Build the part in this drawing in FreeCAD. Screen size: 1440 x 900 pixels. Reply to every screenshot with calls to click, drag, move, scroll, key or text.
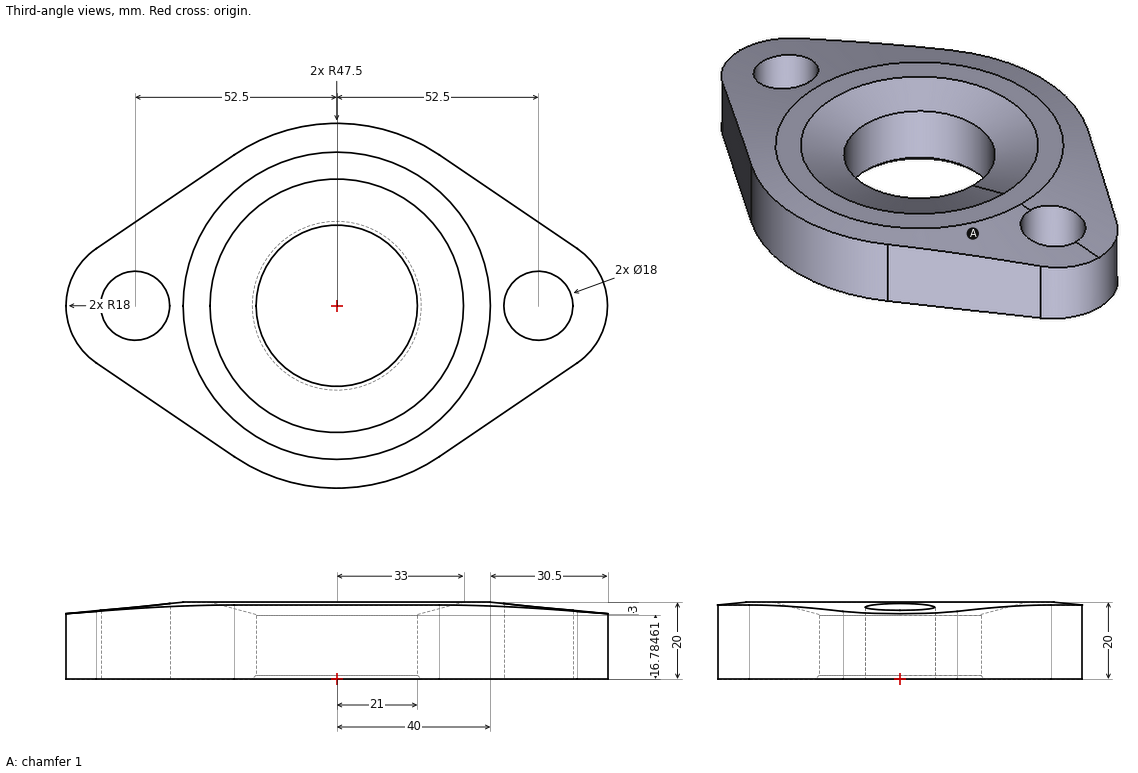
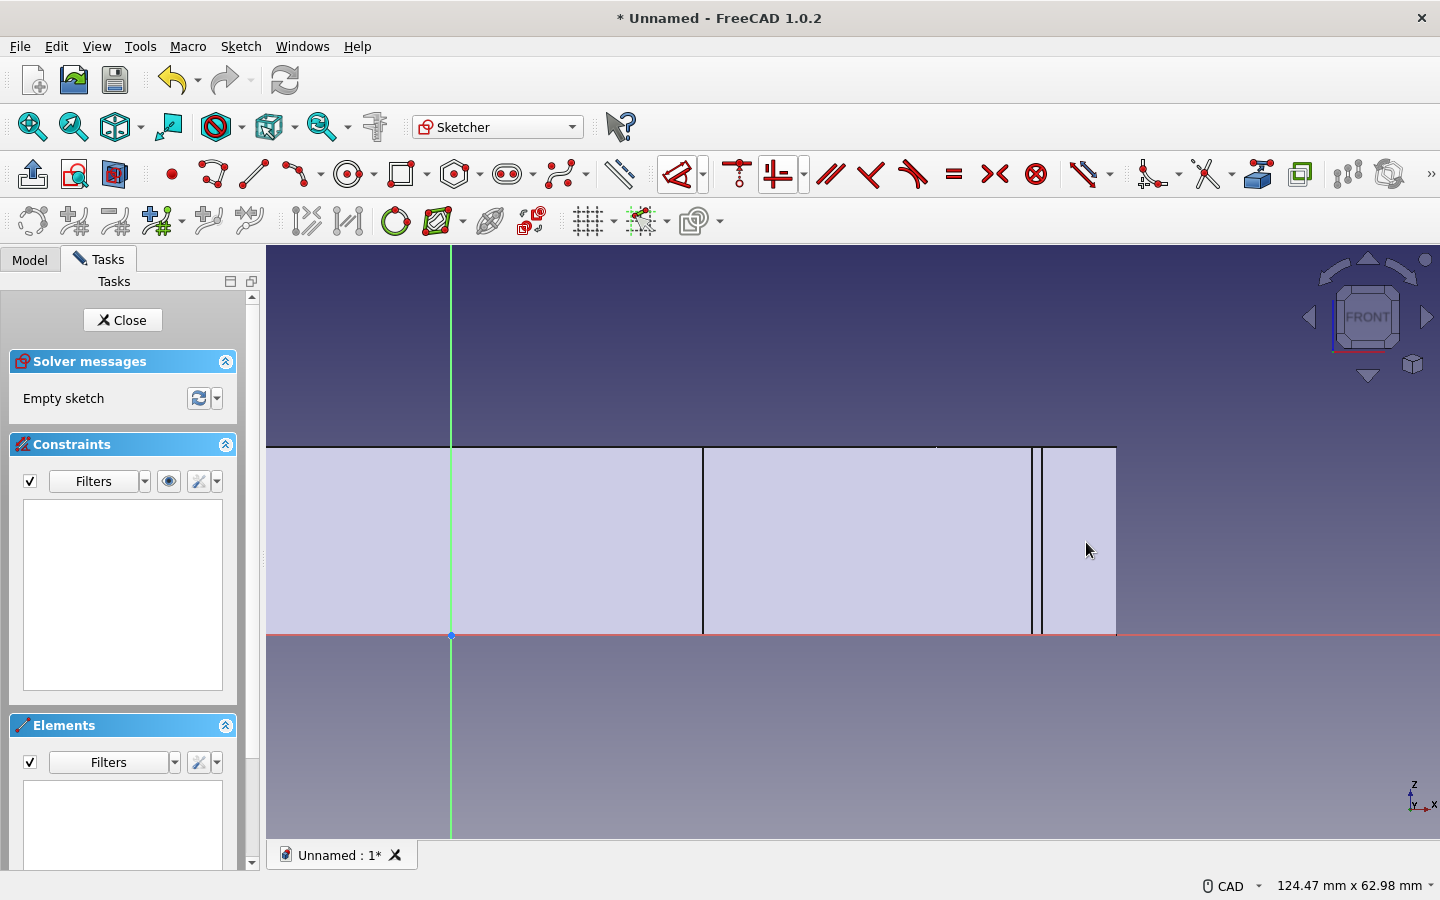
key(g)
key(m)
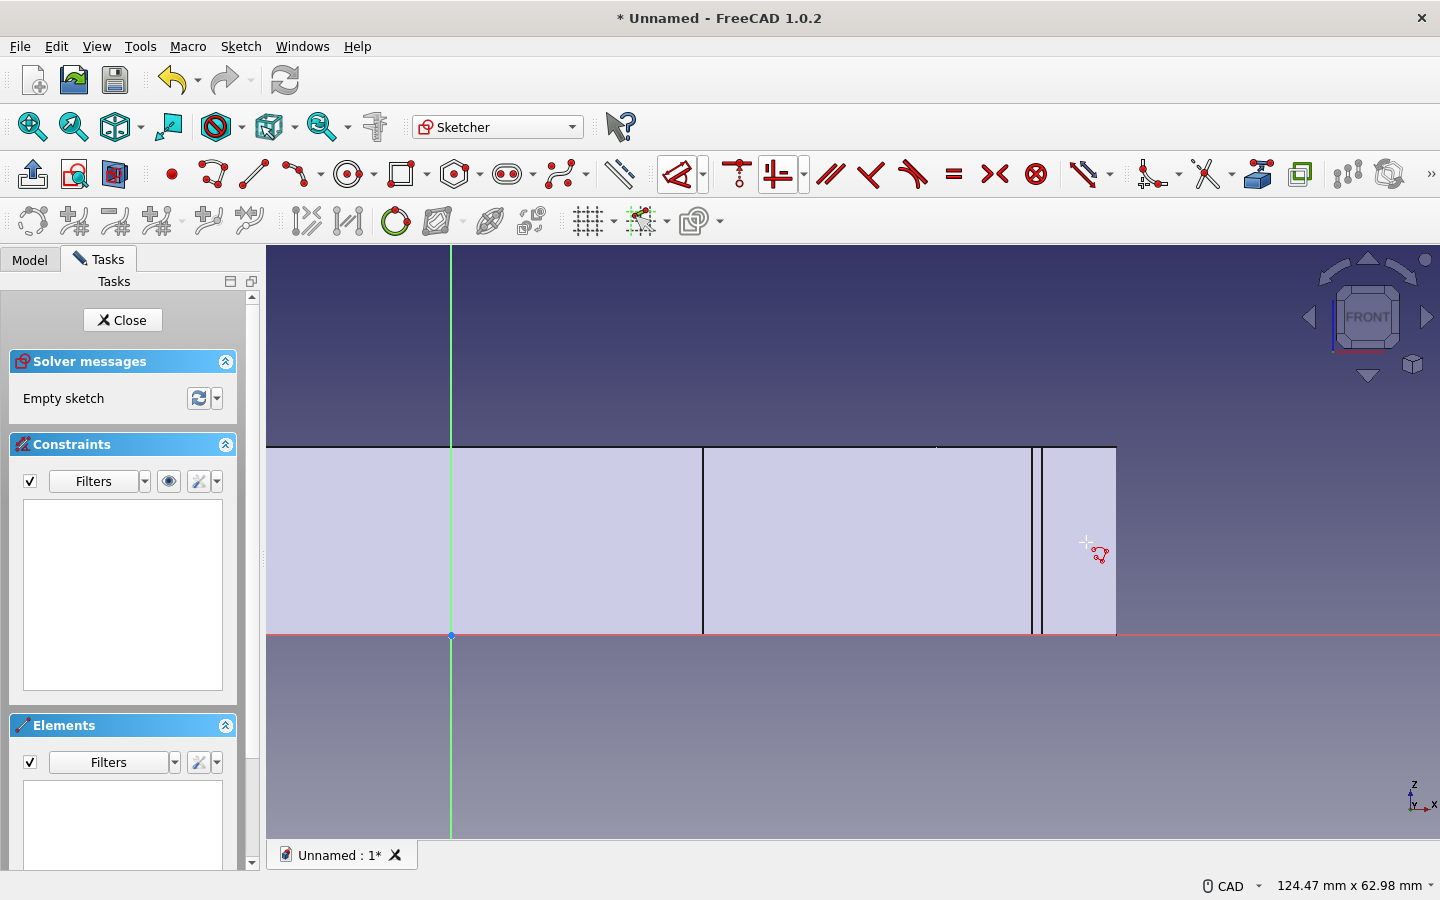
click(451, 635)
click(460, 447)
click(763, 447)
click(650, 477)
click(650, 626)
click(451, 635)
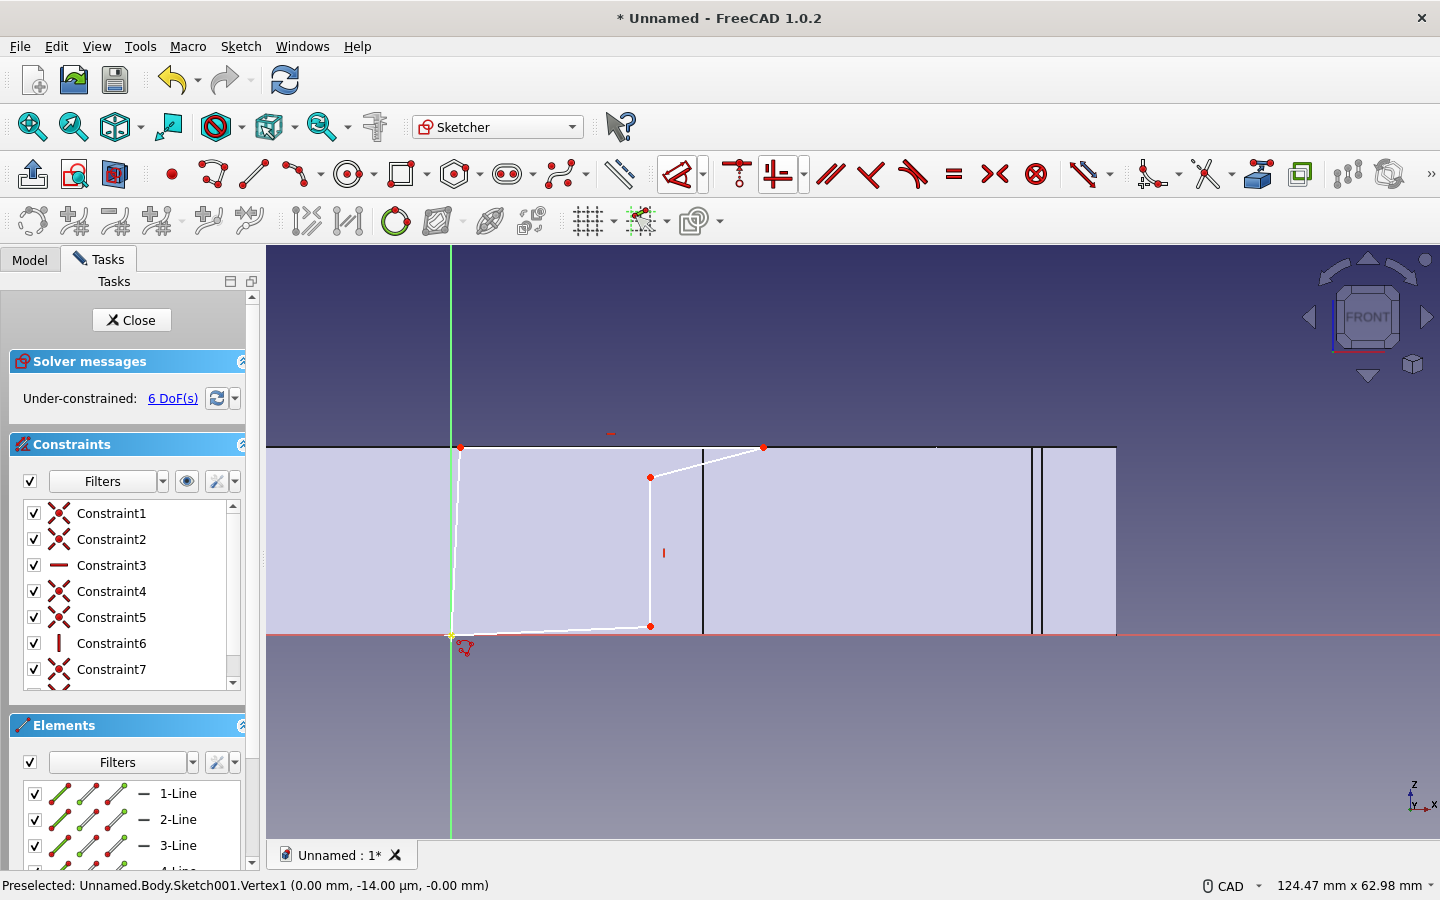
click(829, 447)
click(1116, 447)
click(1116, 475)
click(829, 448)
key(Escape)
key(Escape)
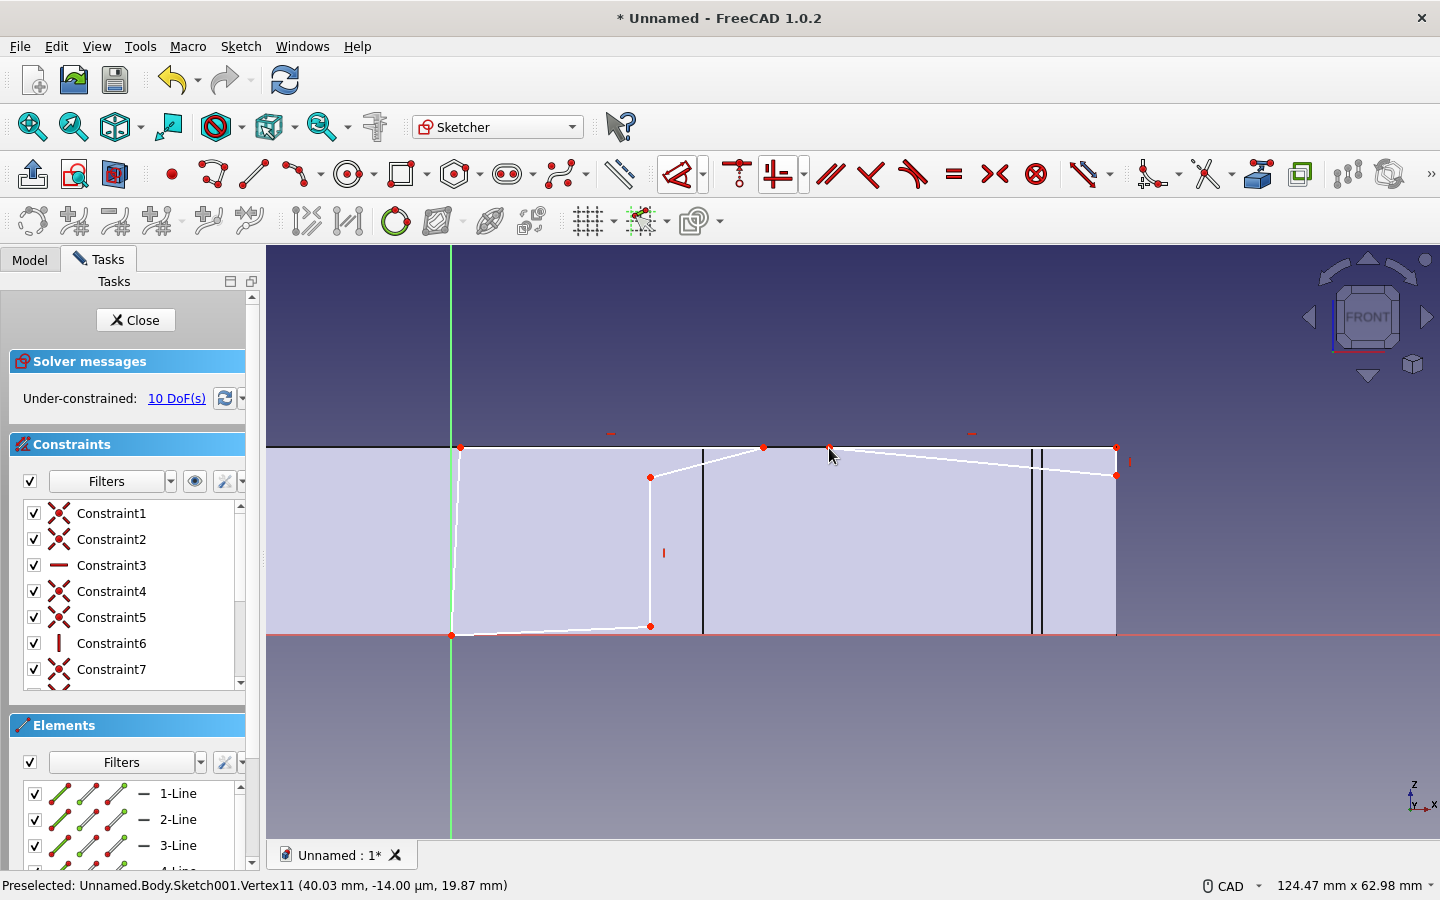
click(454, 579)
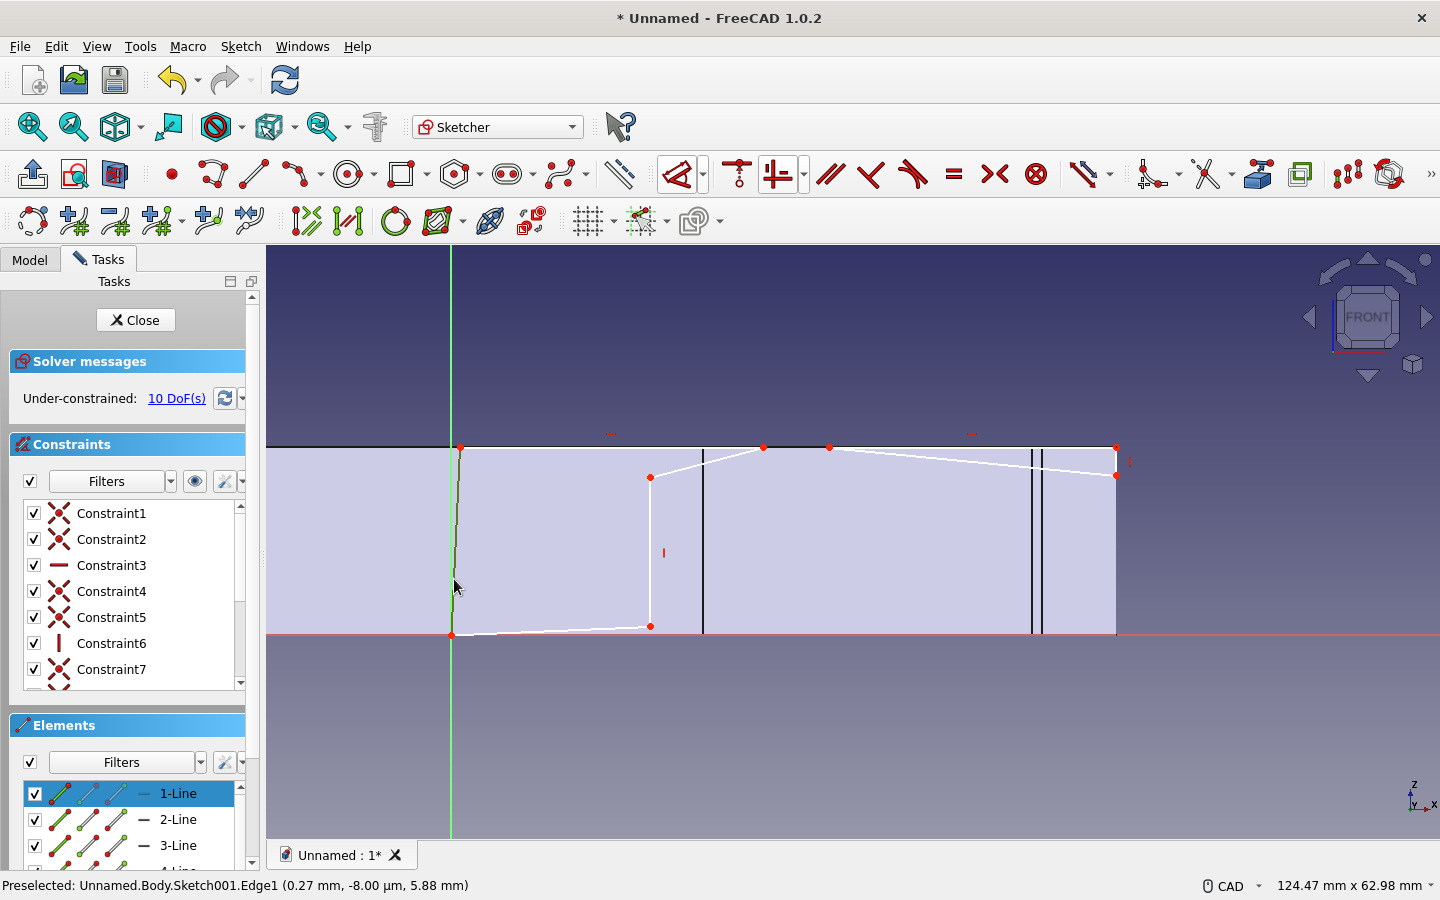
key(v)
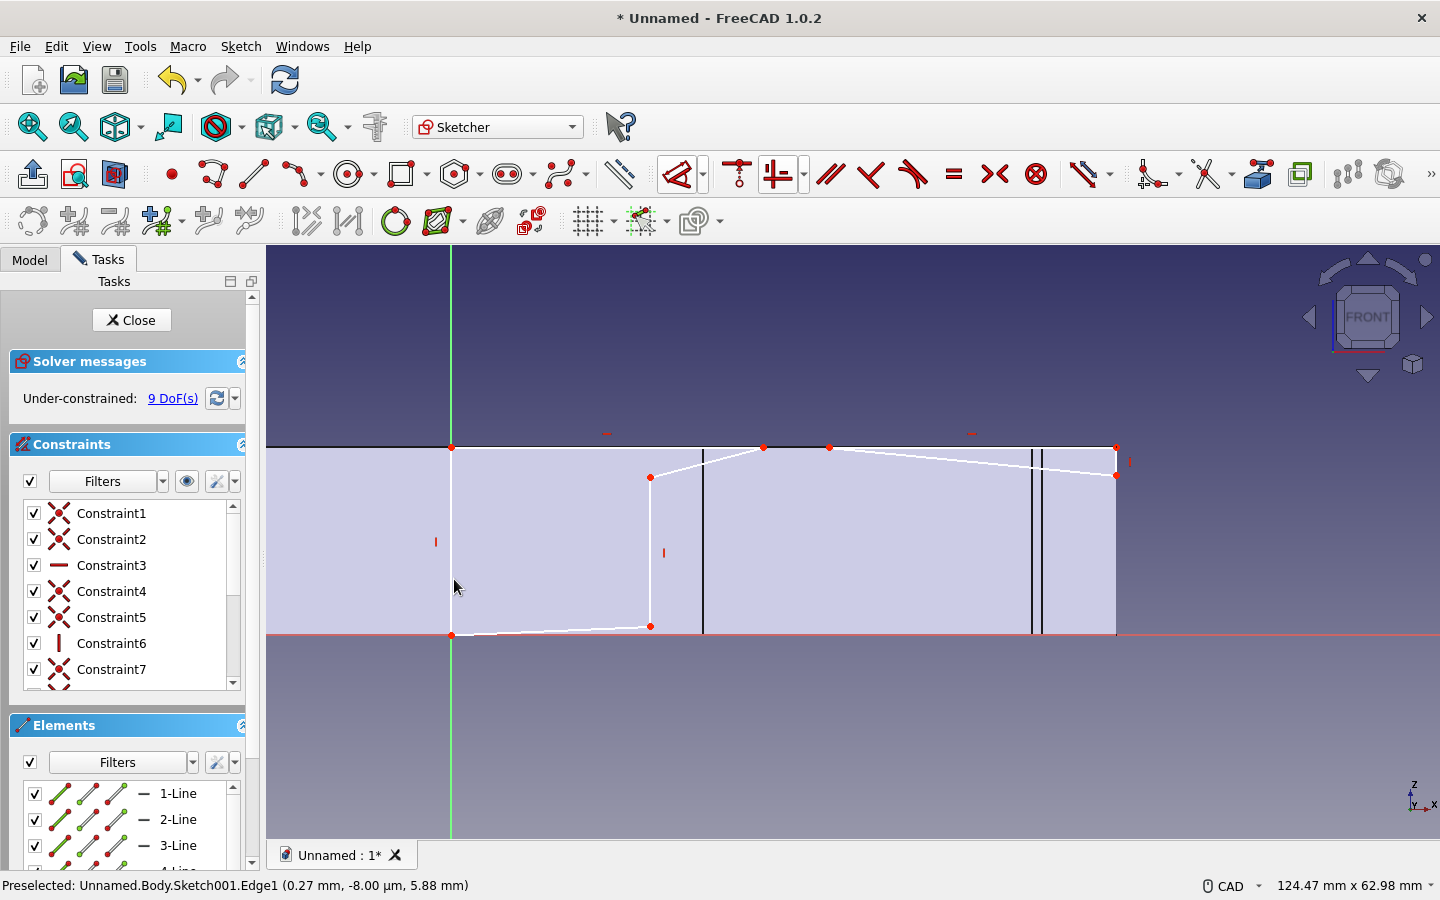
click(511, 633)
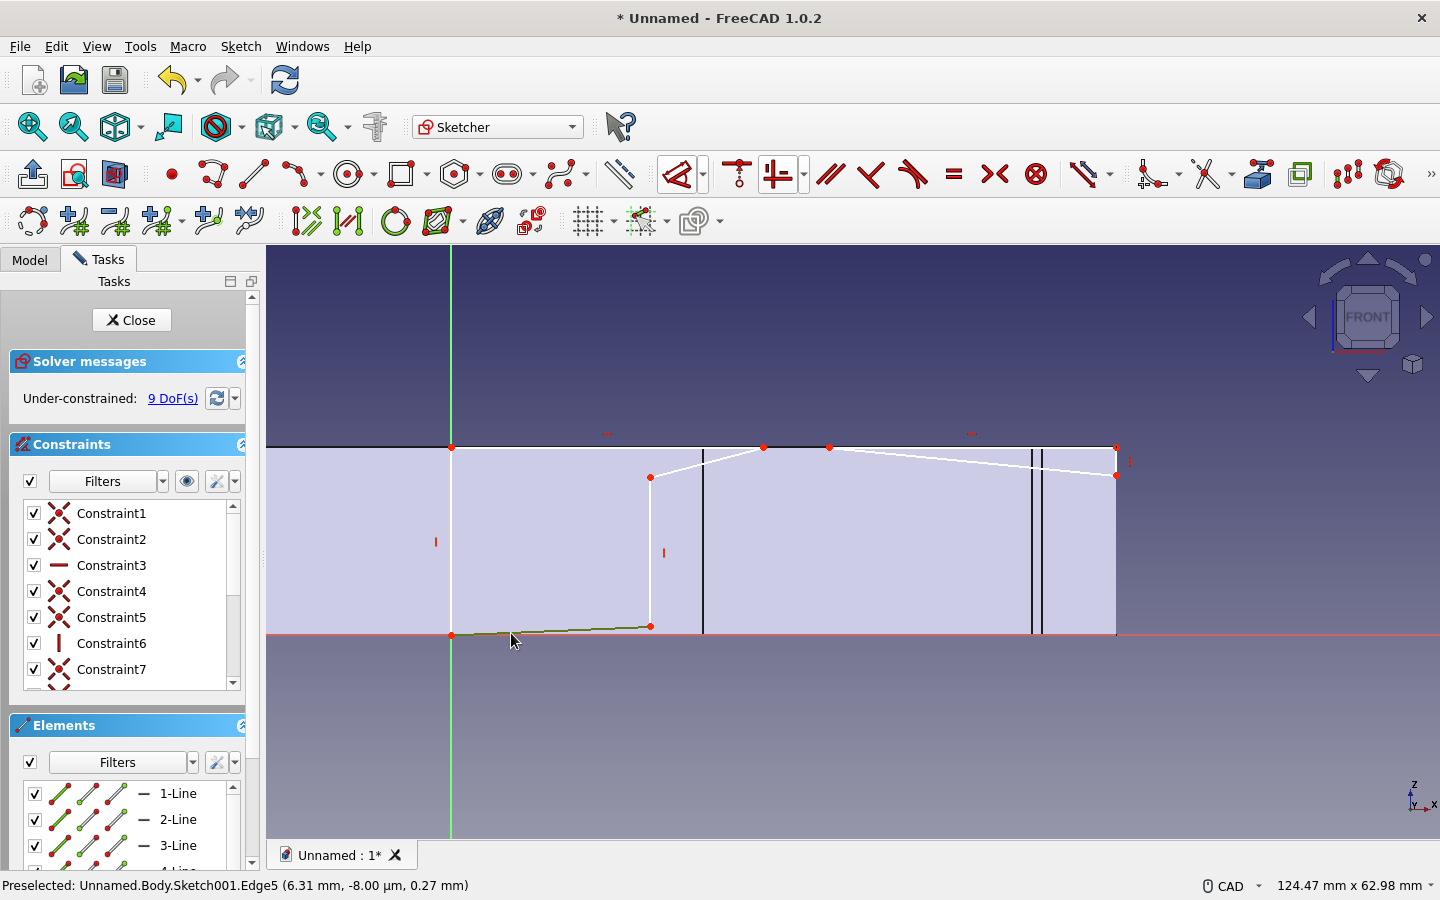
key(h)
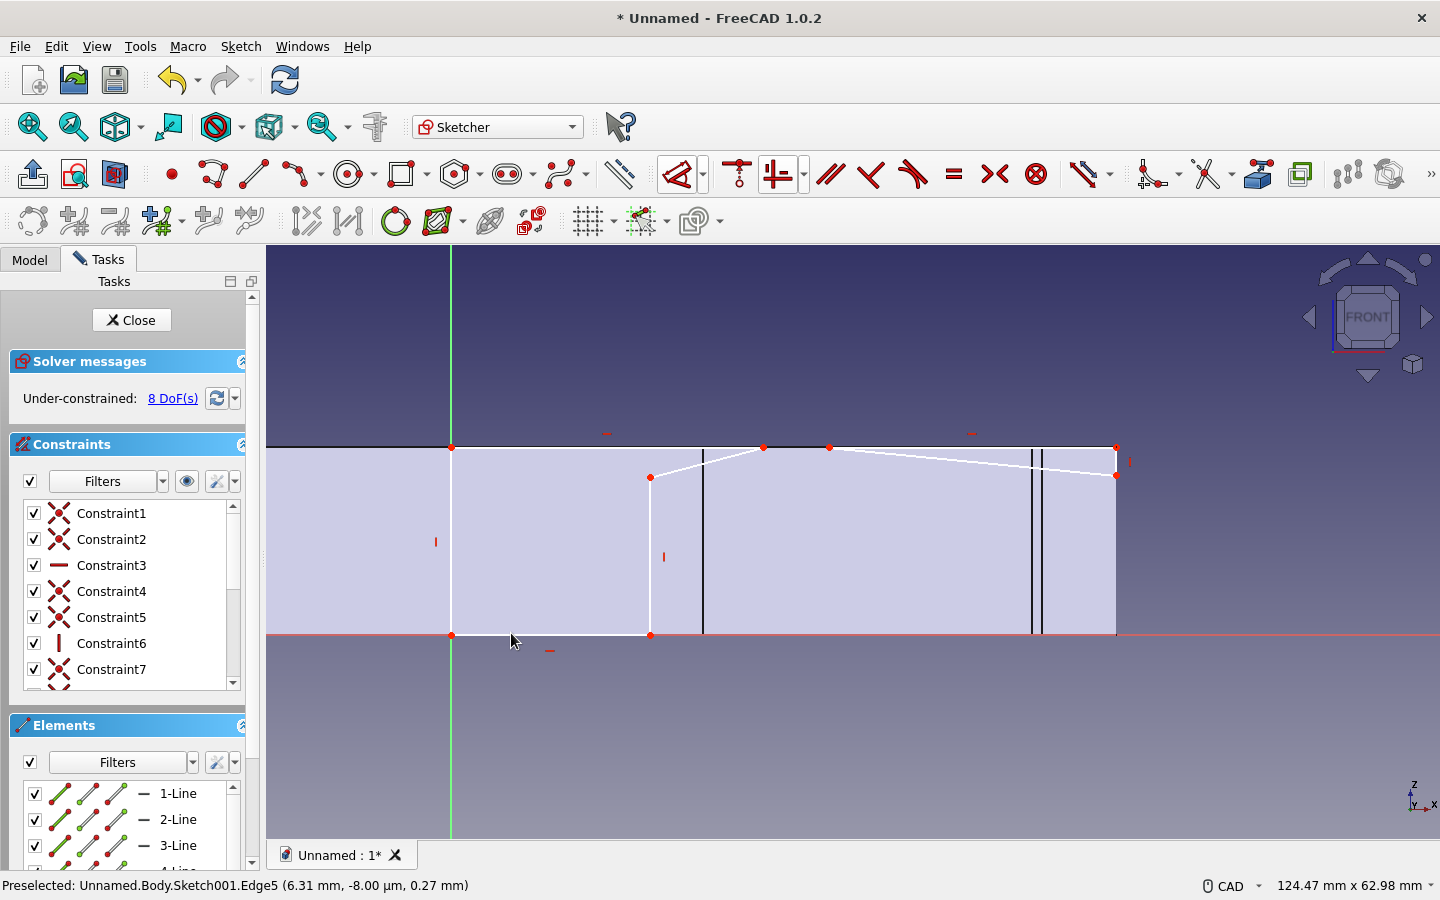
key(d)